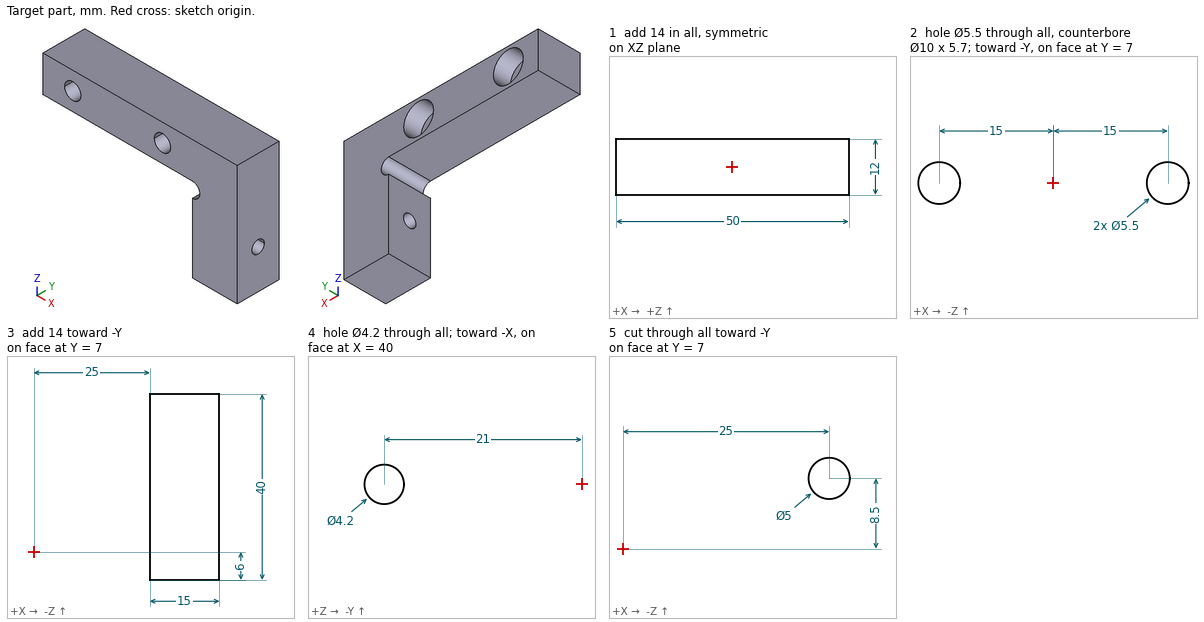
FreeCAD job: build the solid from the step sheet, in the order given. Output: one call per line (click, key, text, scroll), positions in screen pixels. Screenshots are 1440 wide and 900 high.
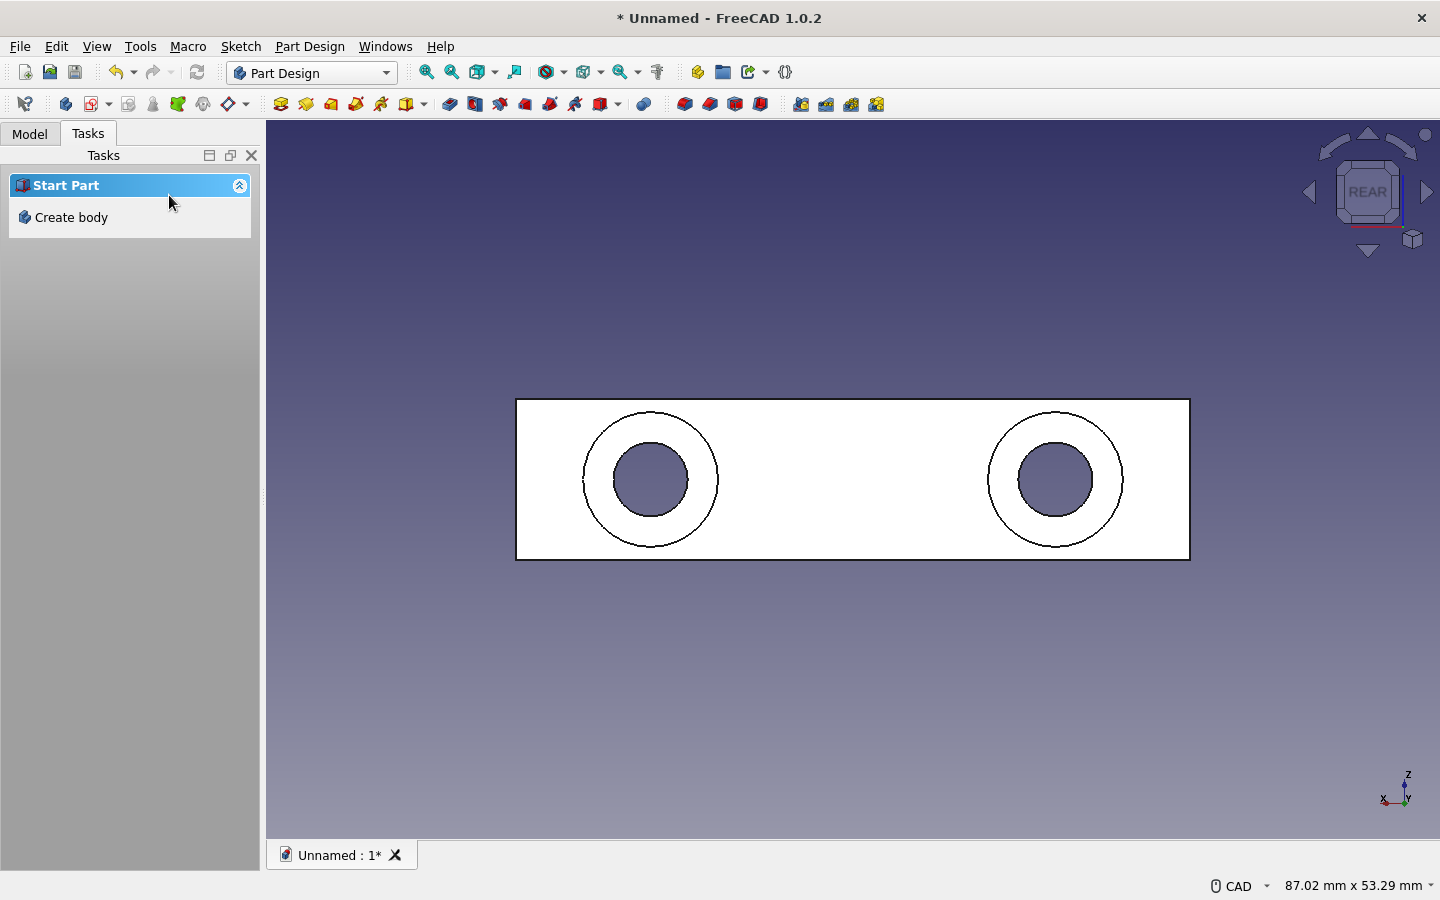
click(853, 479)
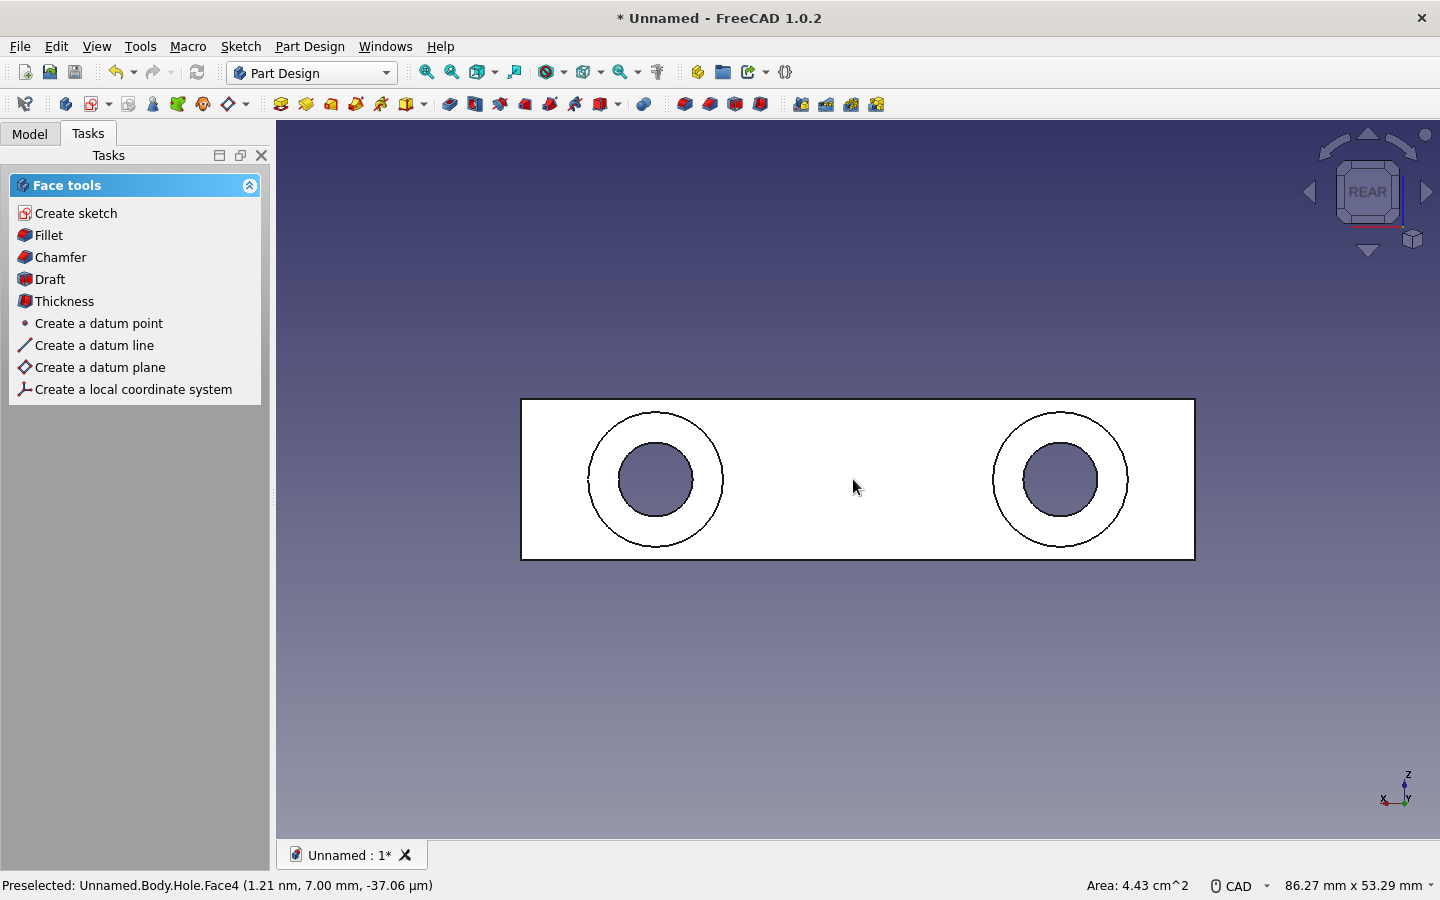
click(90, 104)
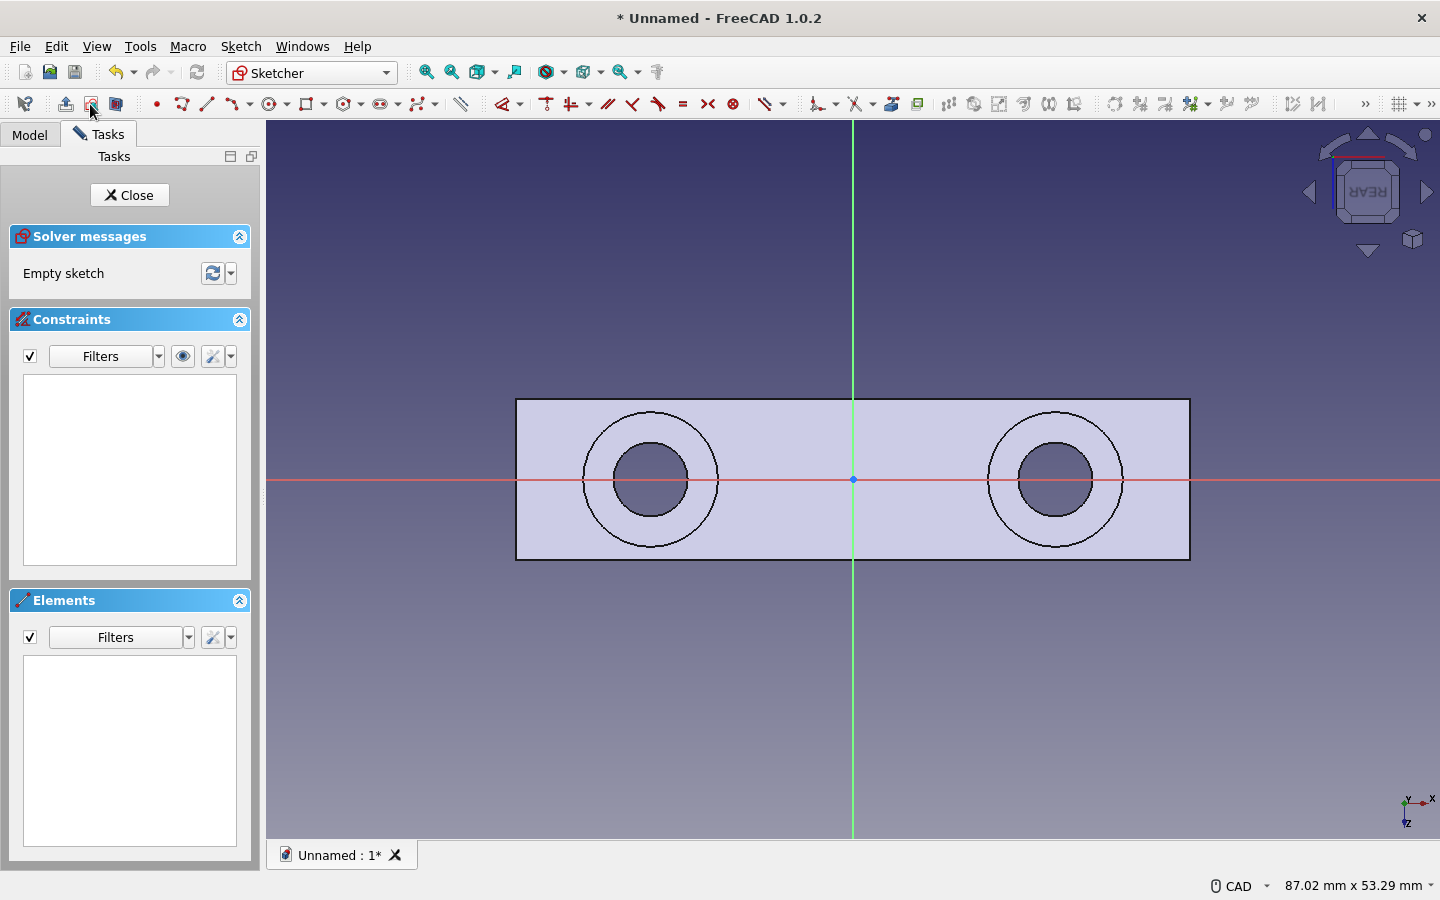
scroll(294, 811, down, 2)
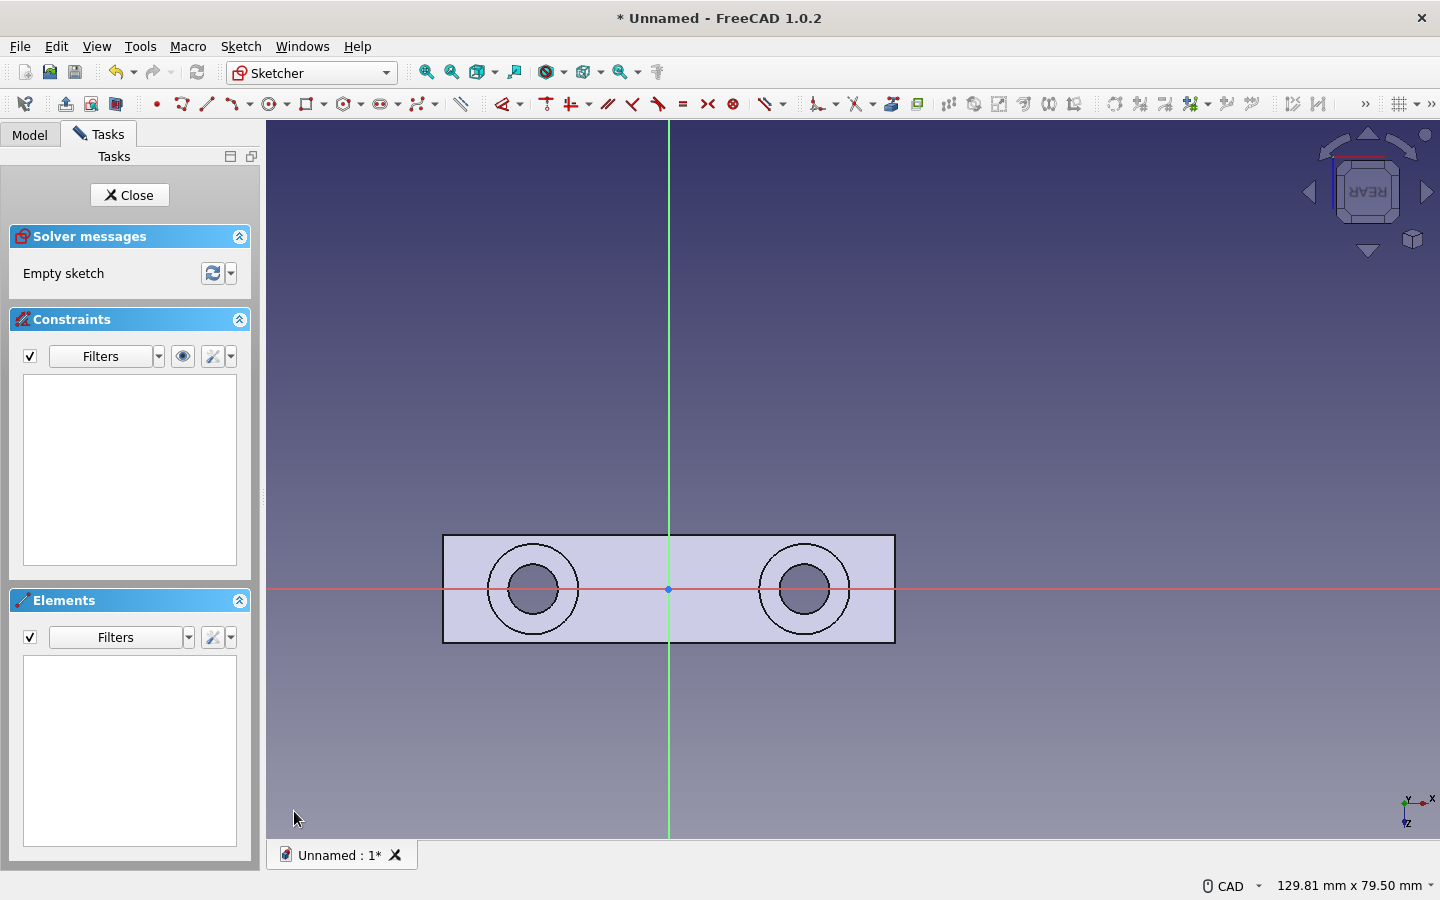
click(306, 104)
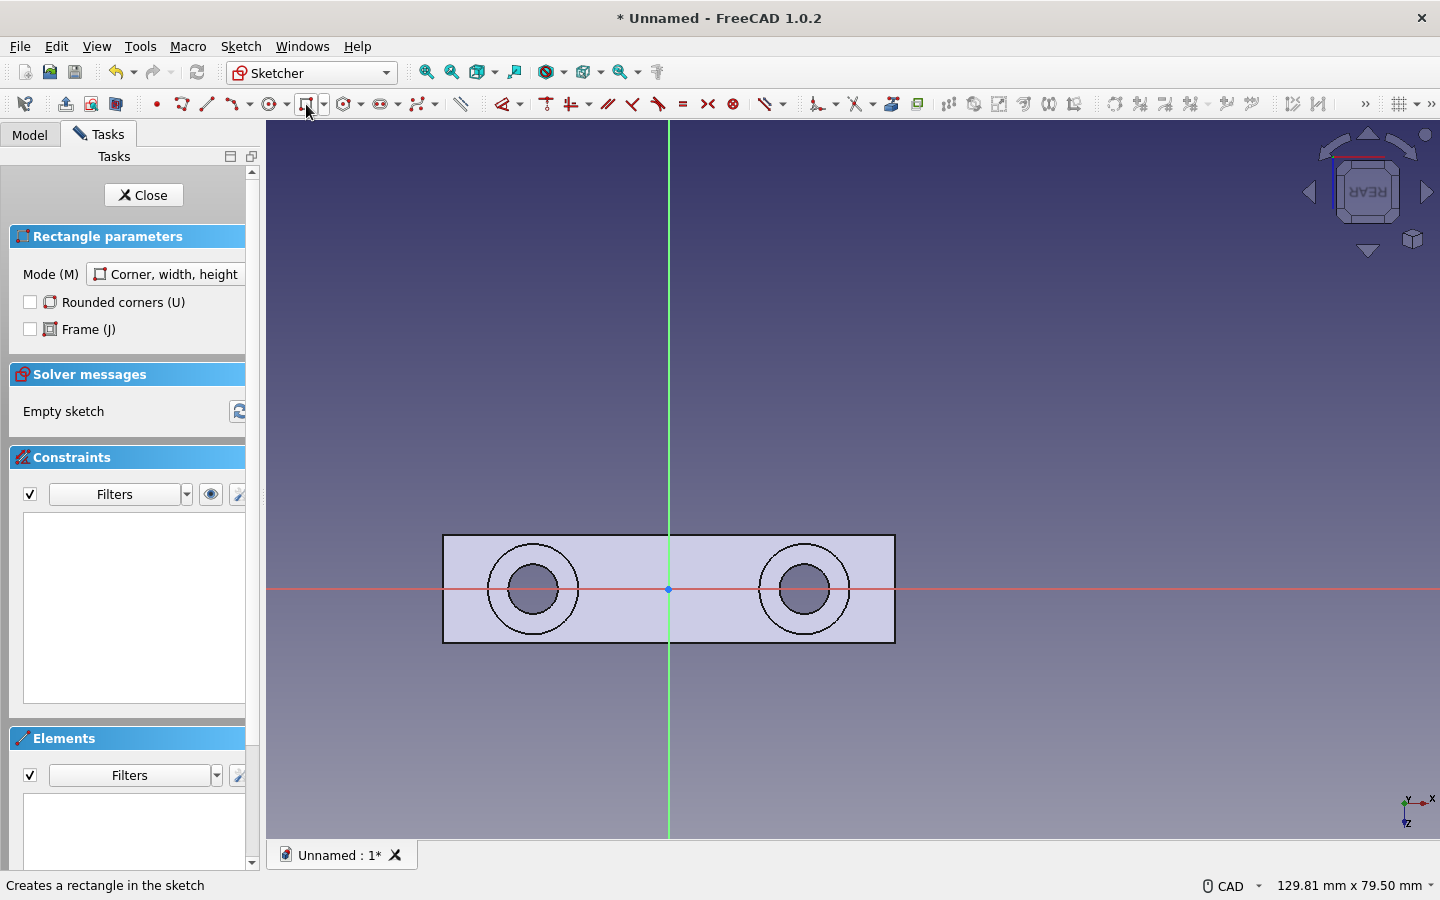
click(895, 282)
move(1030, 643)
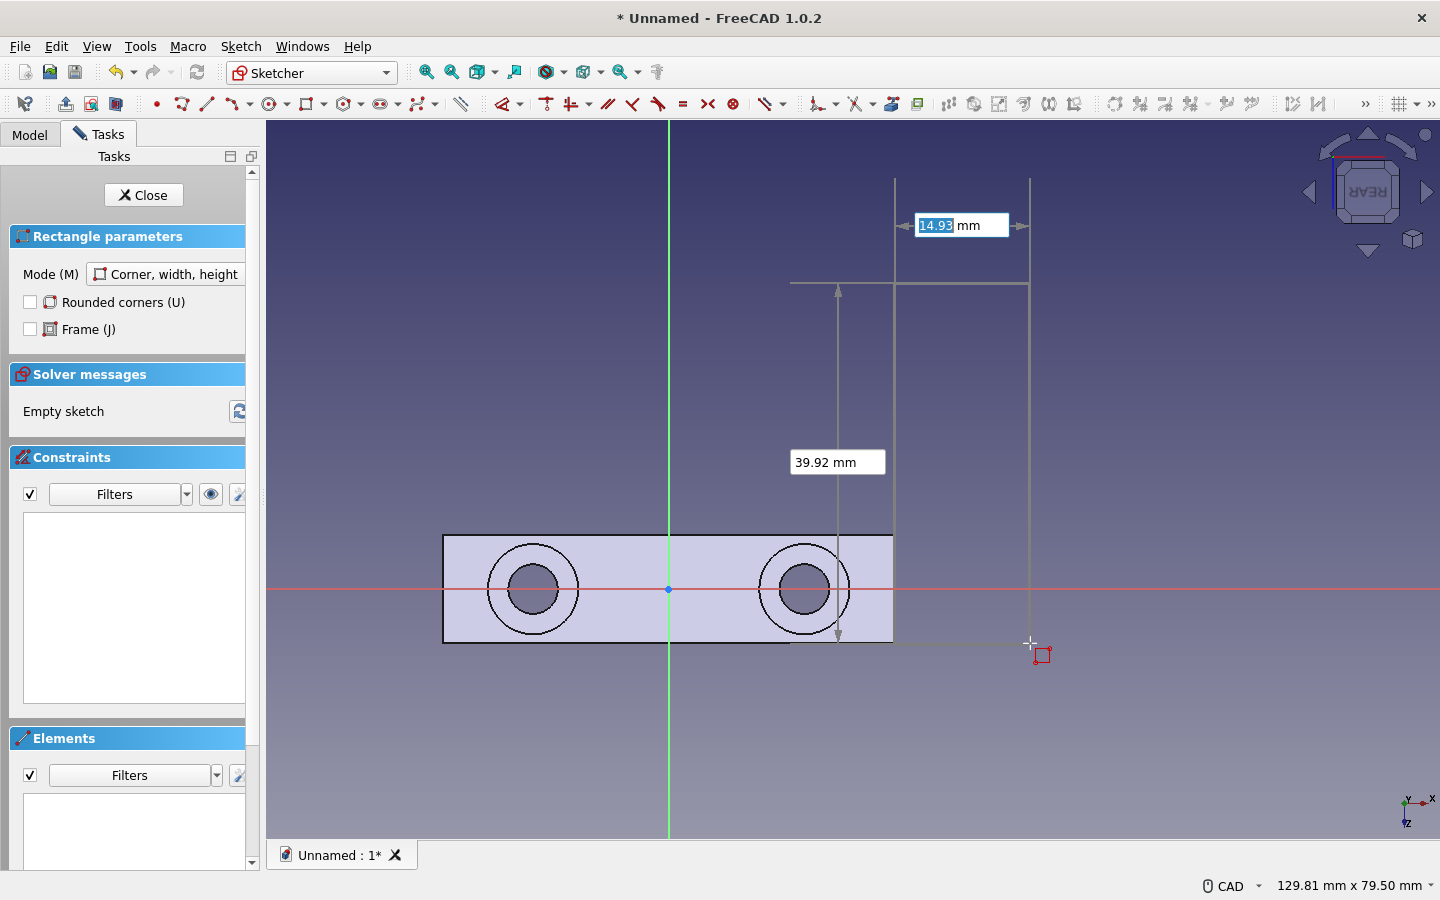
text(15)
key(Tab)
text(40)
key(Return)
key(Escape)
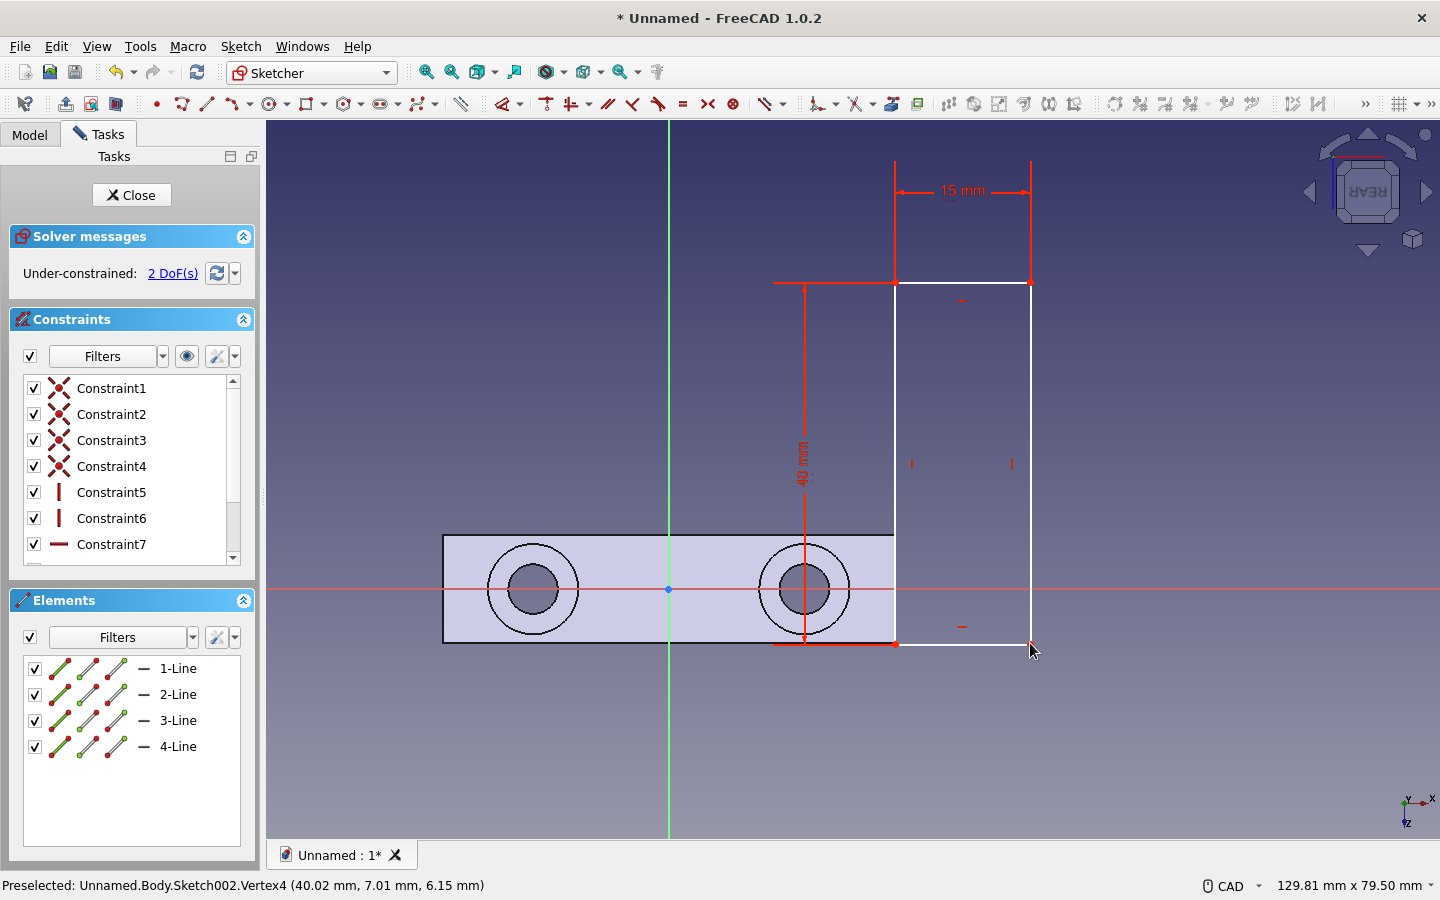
click(502, 104)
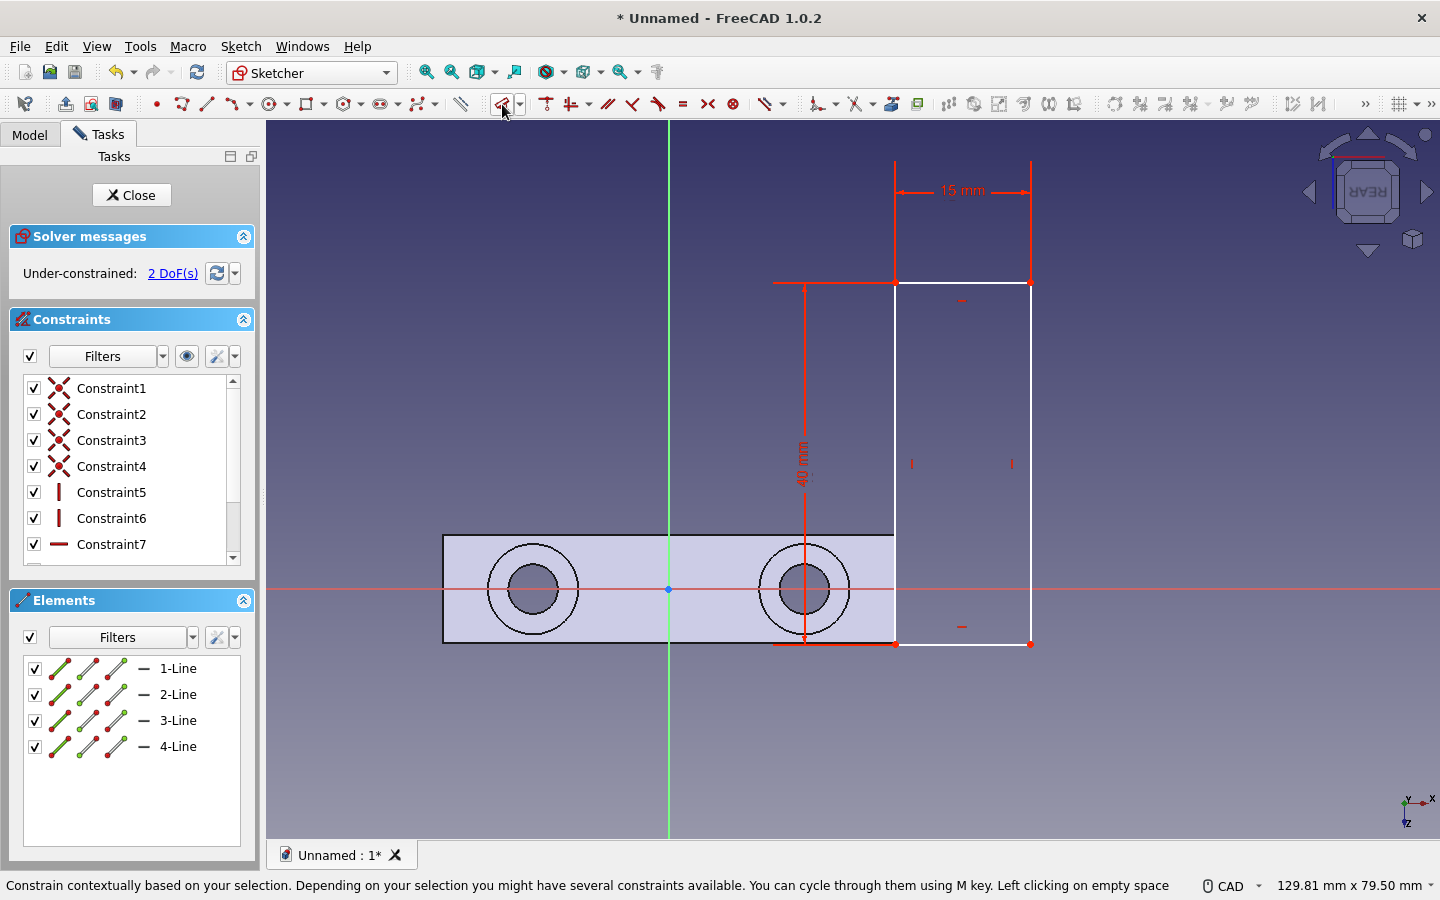
click(895, 645)
click(635, 617)